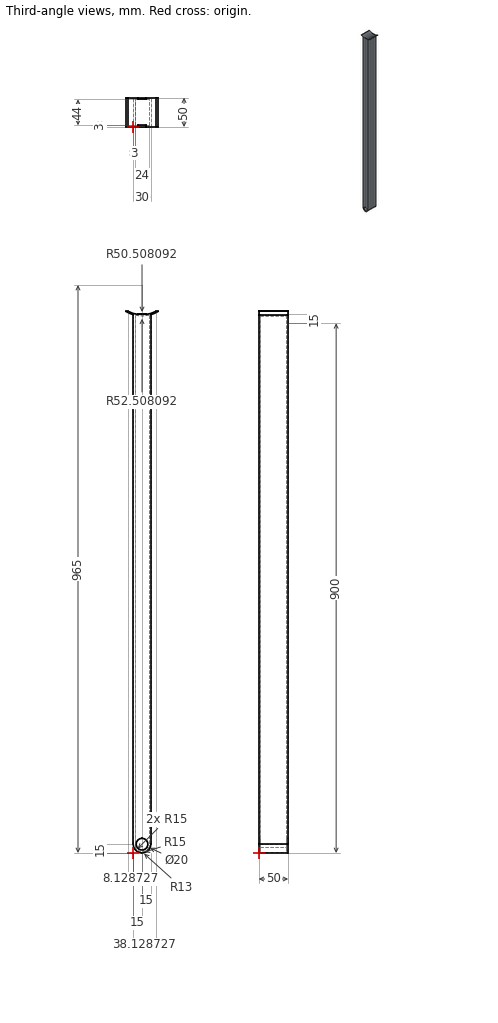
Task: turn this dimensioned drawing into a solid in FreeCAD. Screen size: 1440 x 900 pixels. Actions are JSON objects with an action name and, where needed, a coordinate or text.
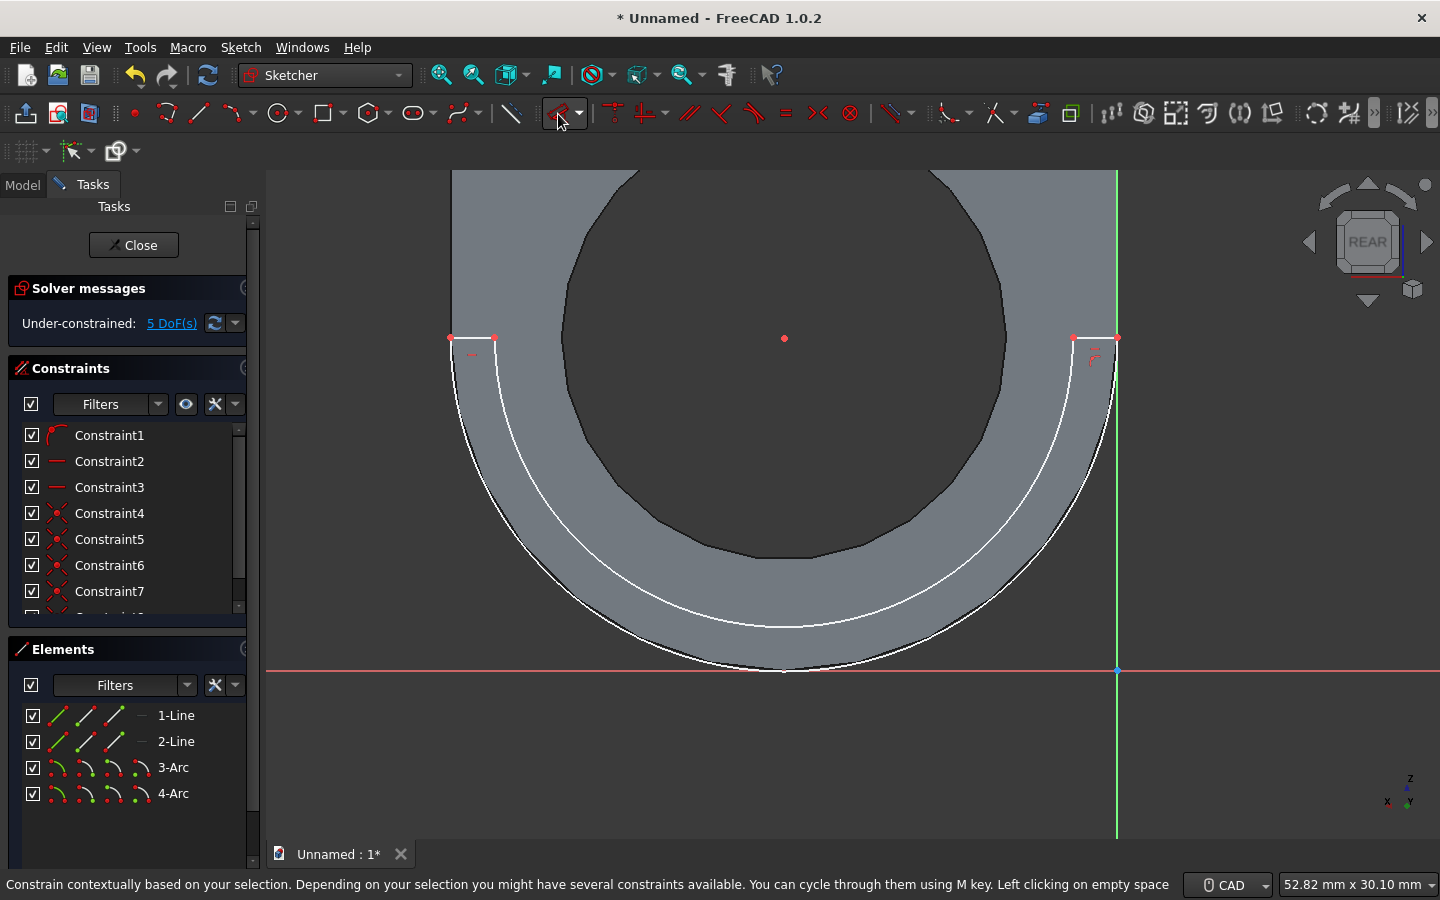
{"action": "left_click", "coordinate": [614, 572]}
{"action": "left_click", "coordinate": [463, 320]}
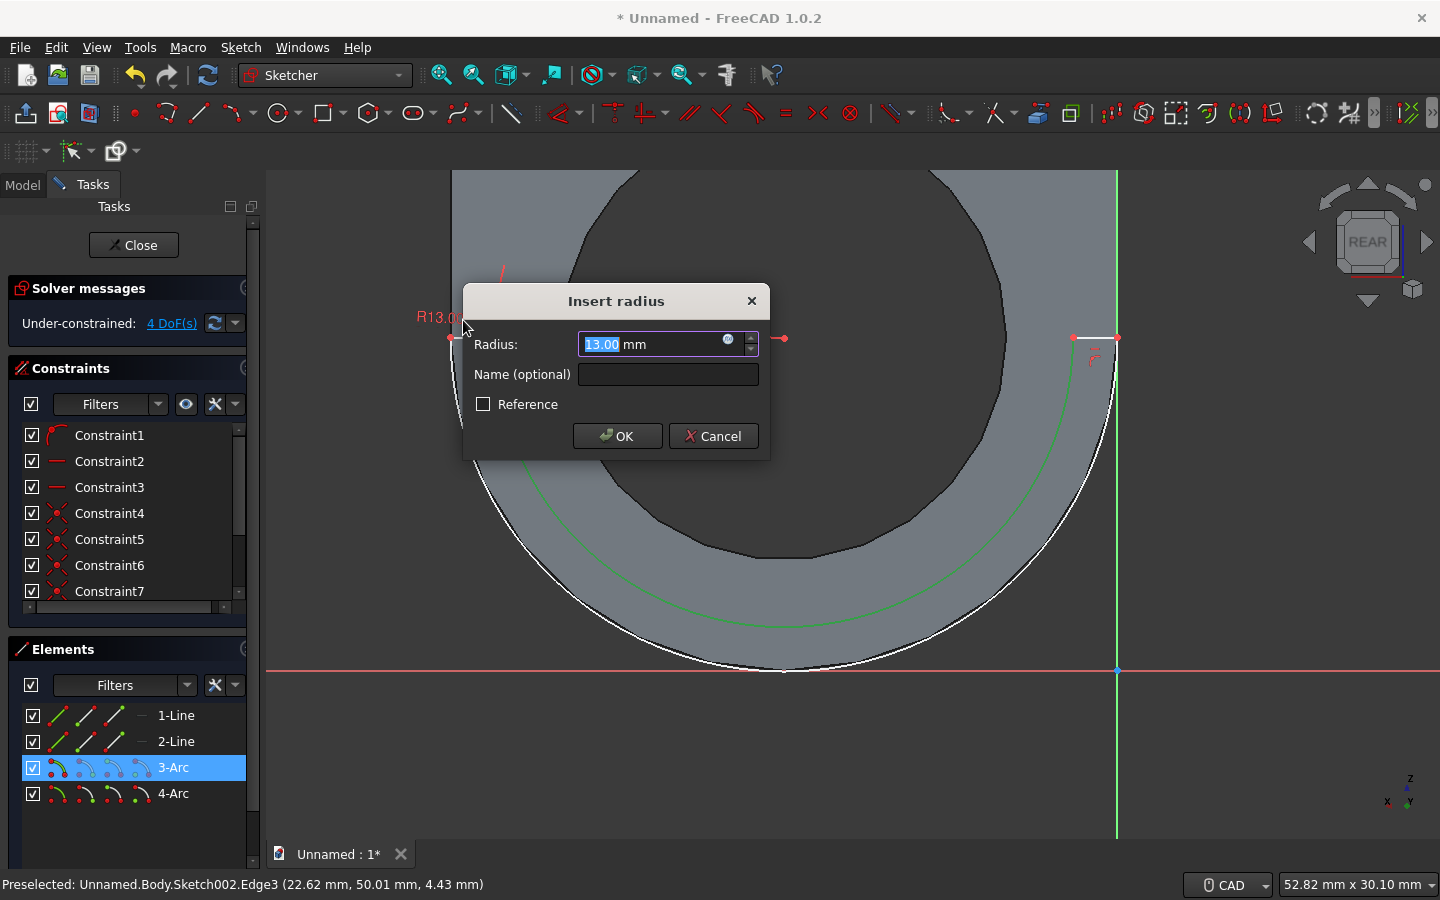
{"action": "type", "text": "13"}
{"action": "key", "text": "Return"}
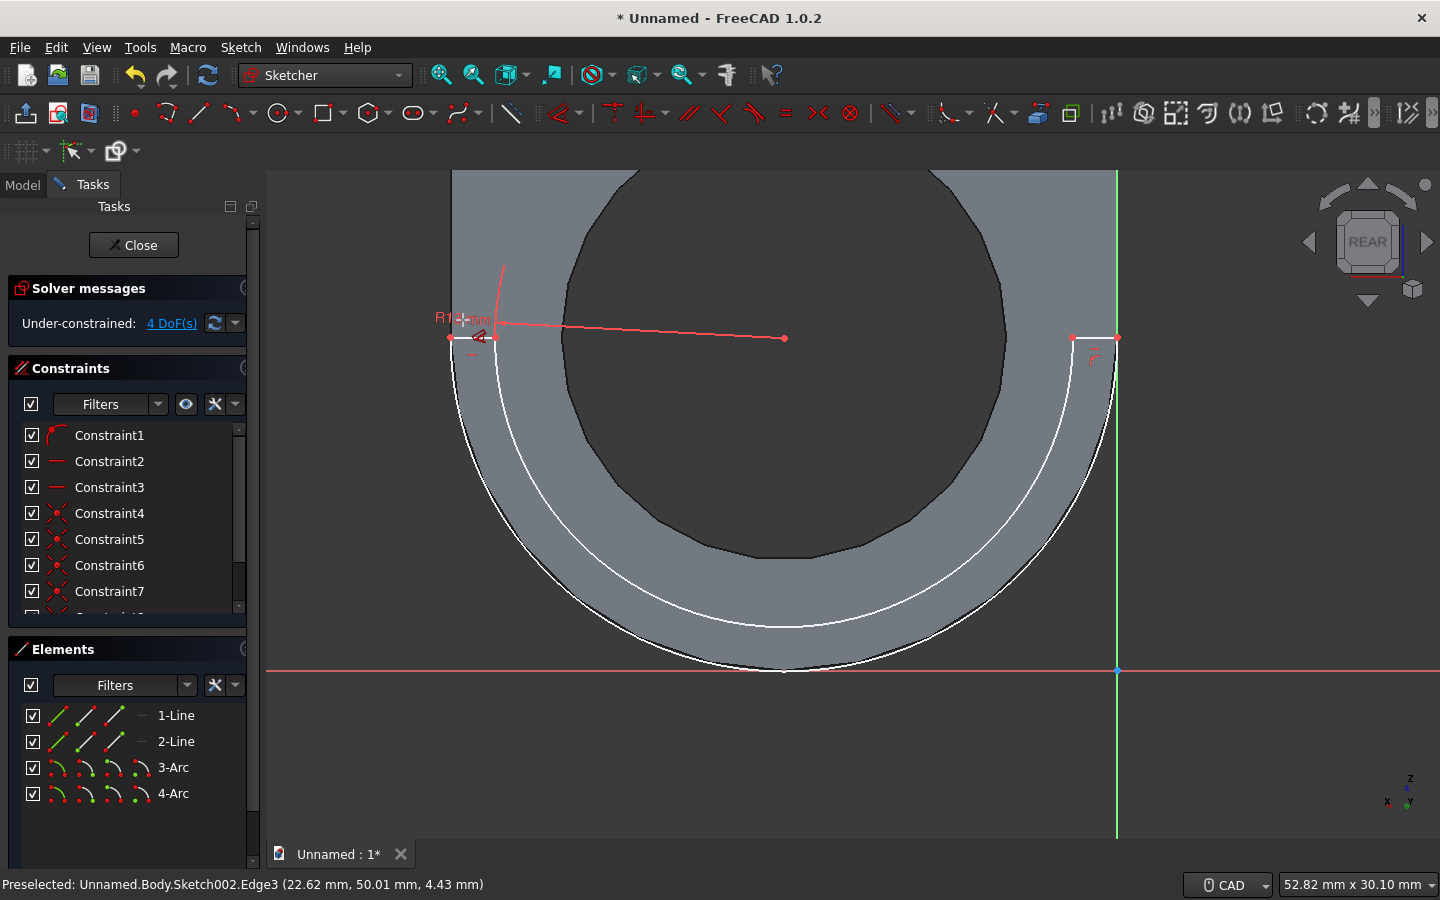
{"action": "left_click", "coordinate": [588, 608]}
{"action": "left_click", "coordinate": [569, 634]}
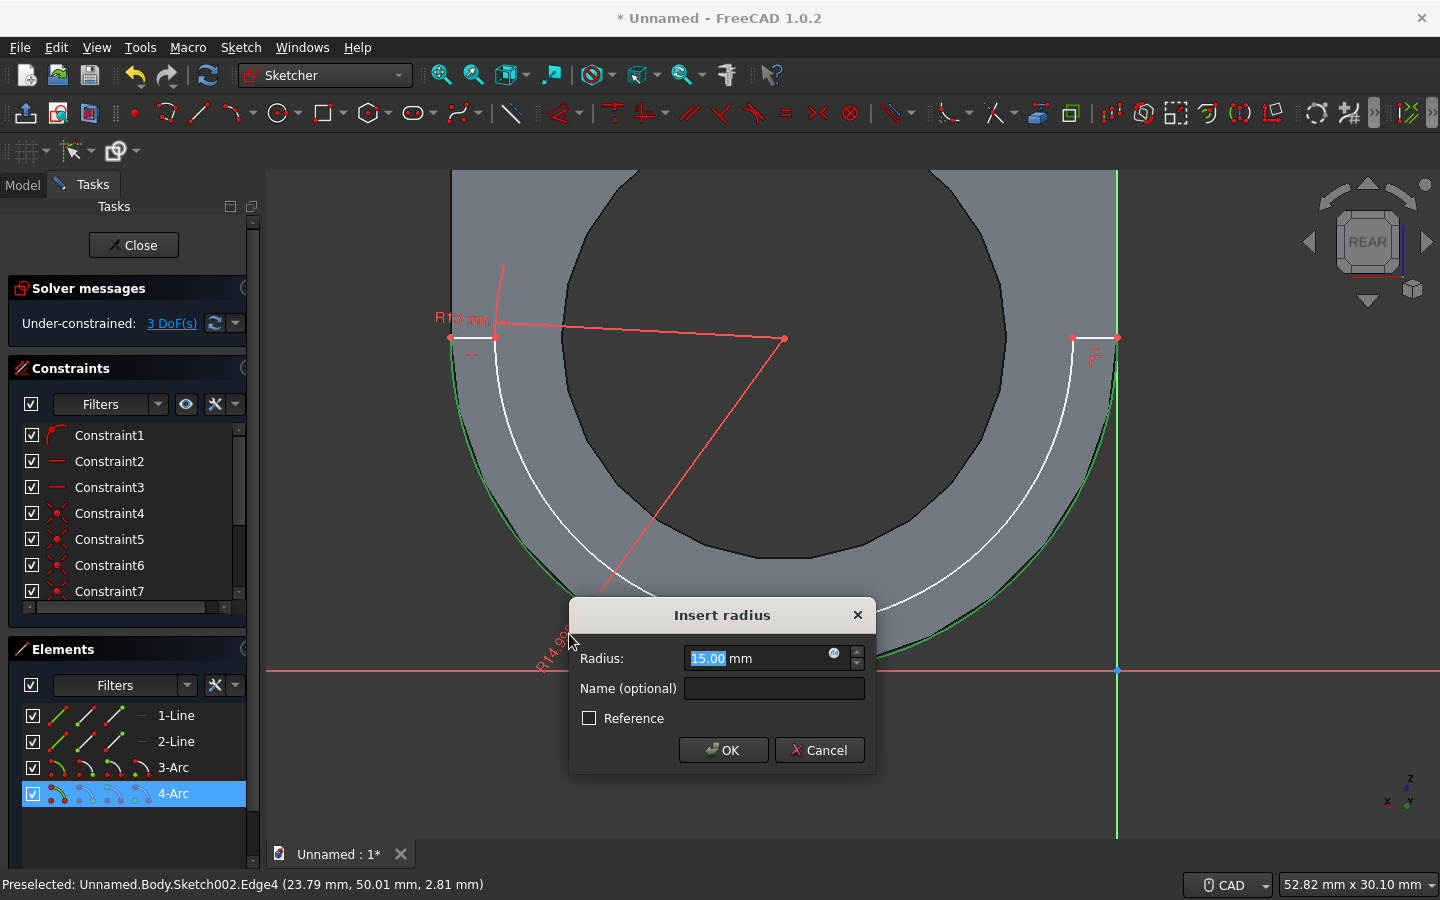
{"action": "type", "text": "15"}
{"action": "key", "text": "Return"}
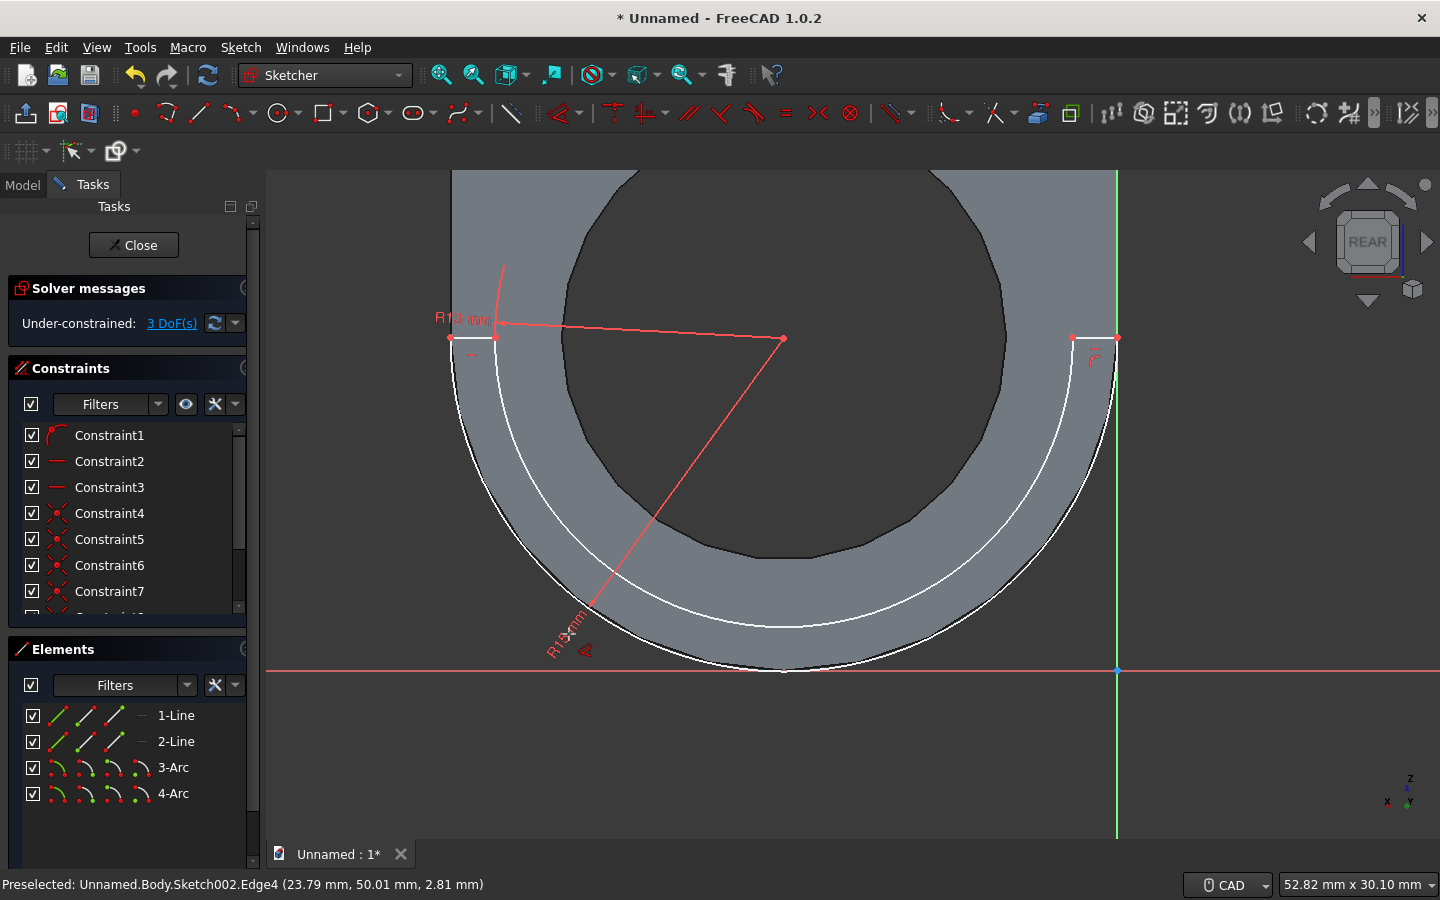
{"action": "left_click", "coordinate": [1117, 338]}
{"action": "left_click", "coordinate": [1151, 504]}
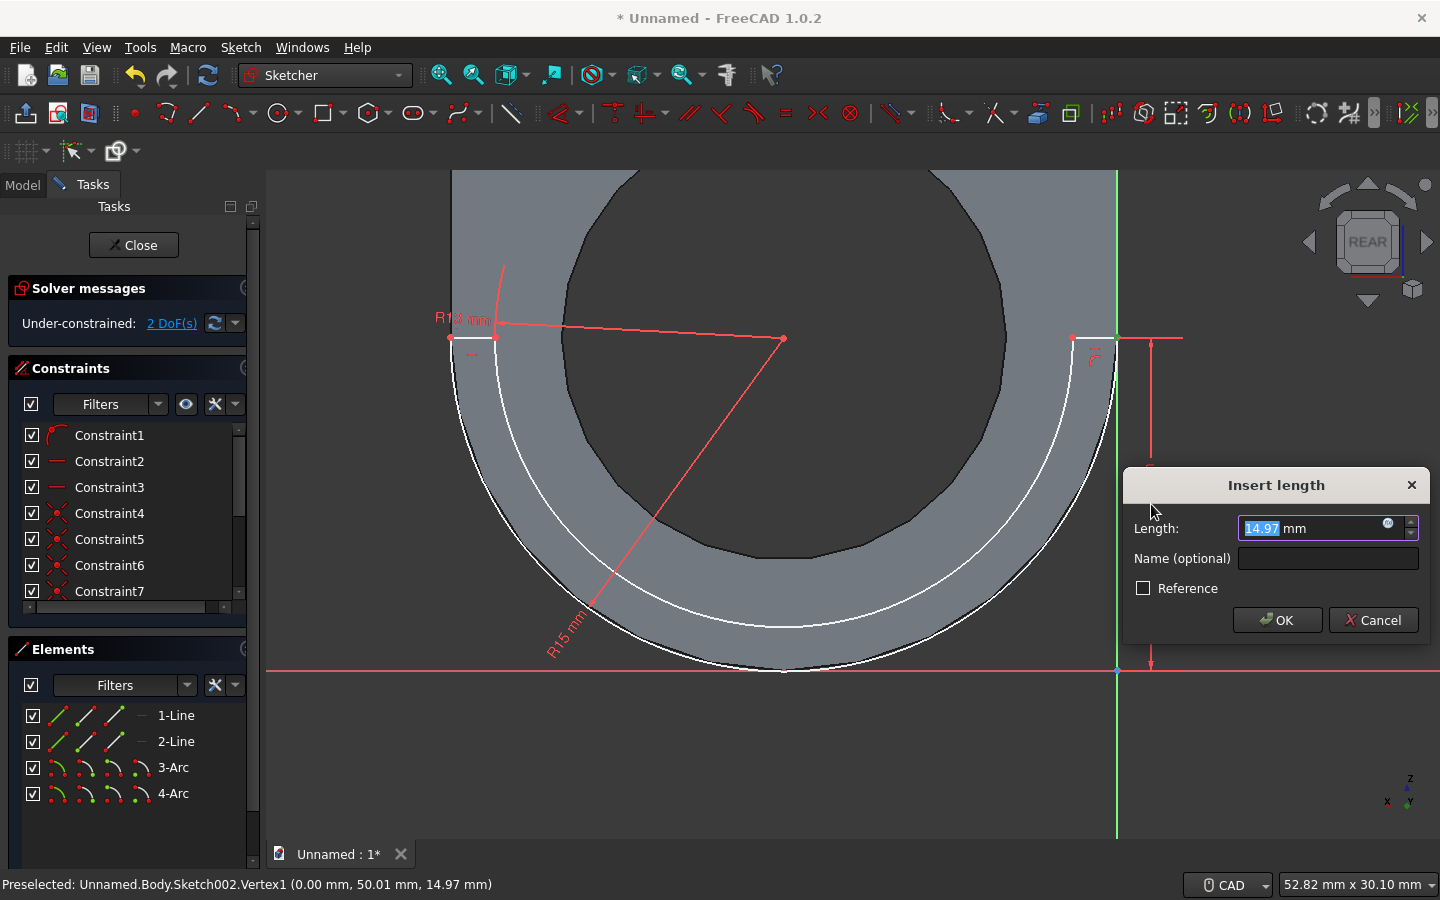
{"action": "type", "text": "15"}
{"action": "key", "text": "Return"}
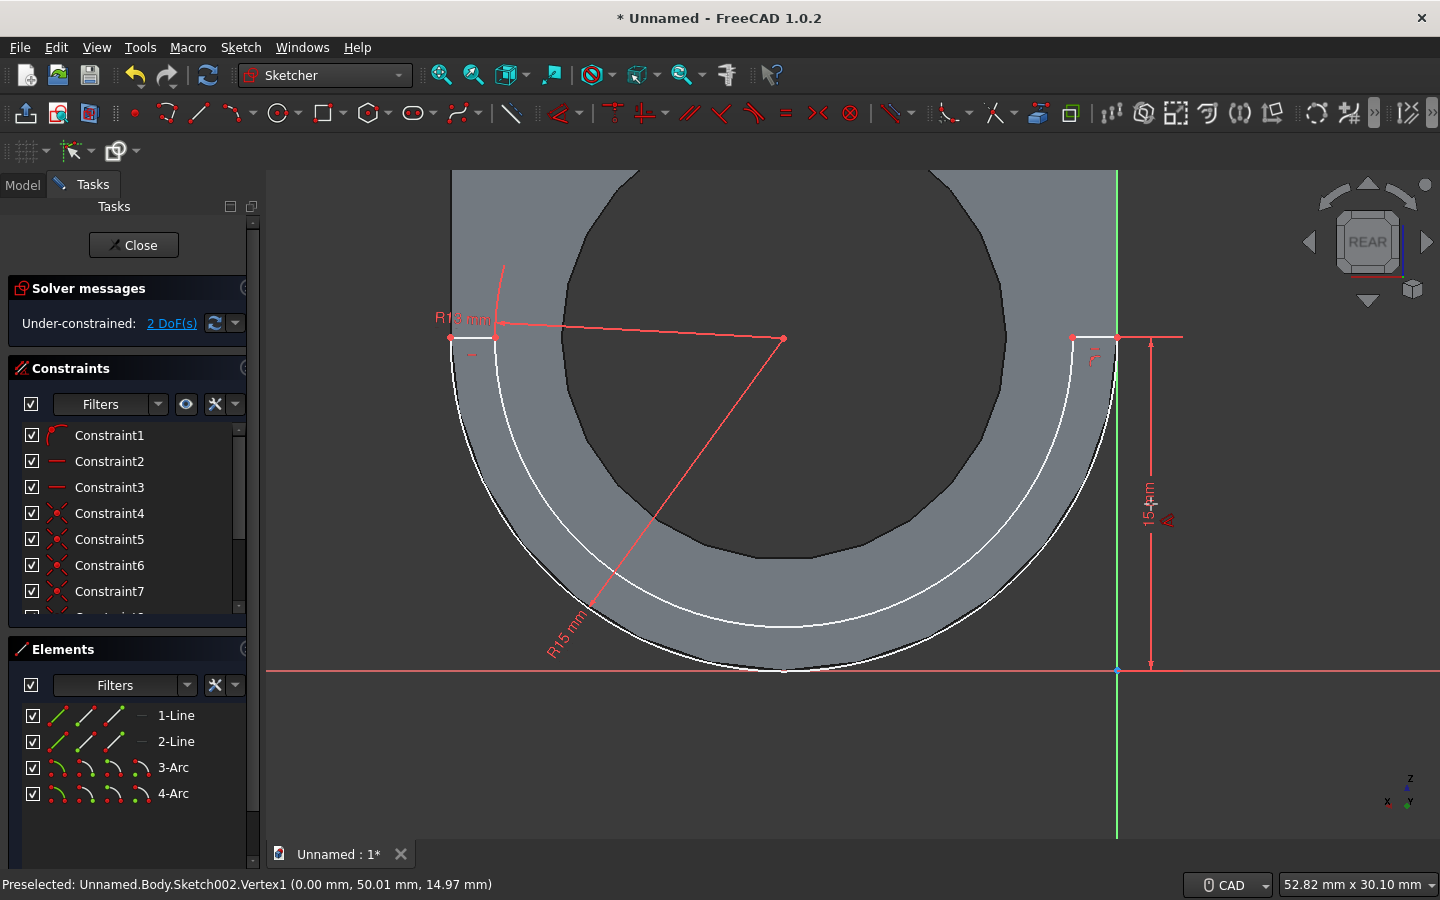
{"action": "left_click", "coordinate": [495, 338]}
{"action": "left_click", "coordinate": [1151, 428]}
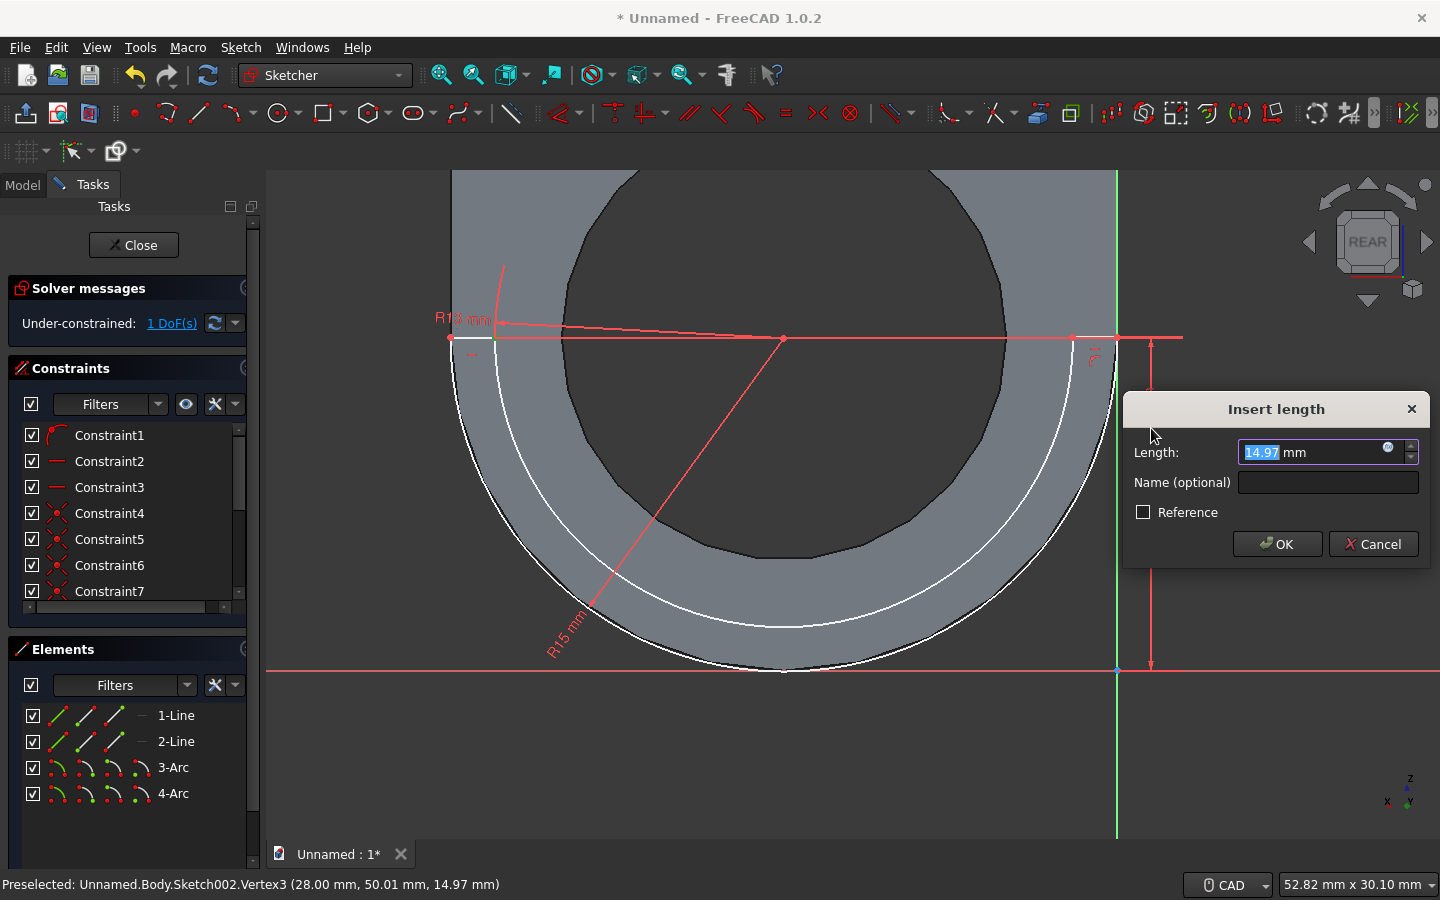
{"action": "type", "text": "15"}
{"action": "key", "text": "Return"}